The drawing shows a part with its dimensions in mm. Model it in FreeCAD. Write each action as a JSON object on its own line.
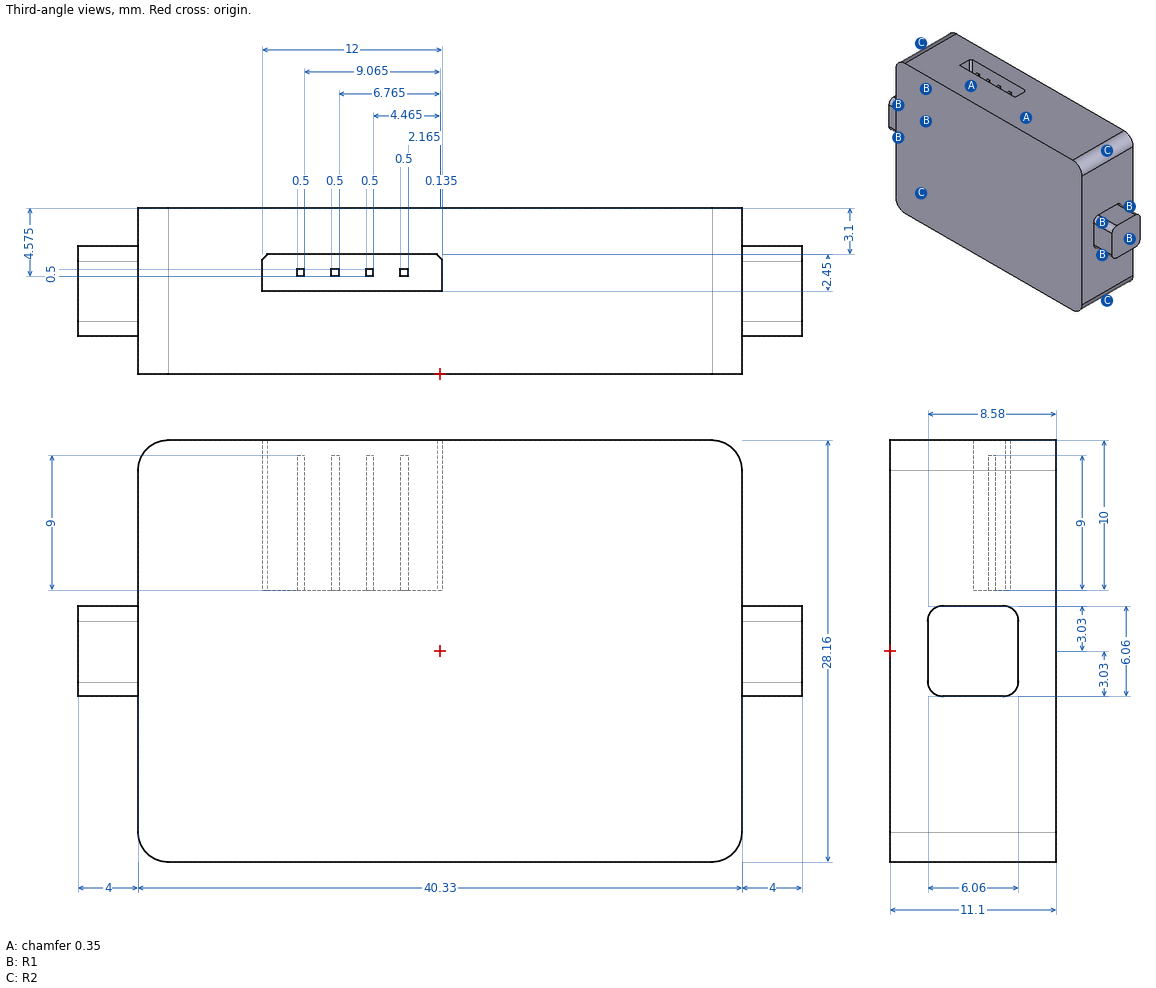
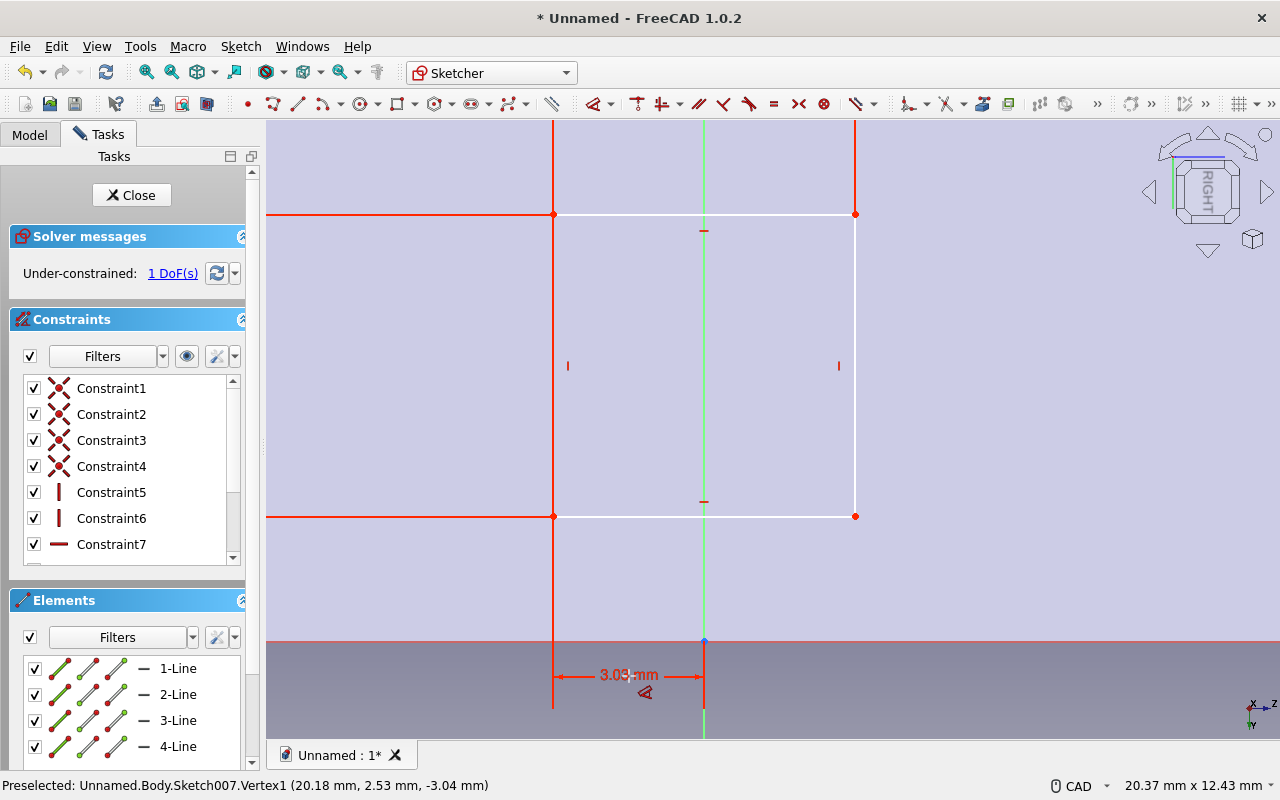
{"action": "left_click", "coordinate": [553, 215]}
{"action": "left_click", "coordinate": [519, 428]}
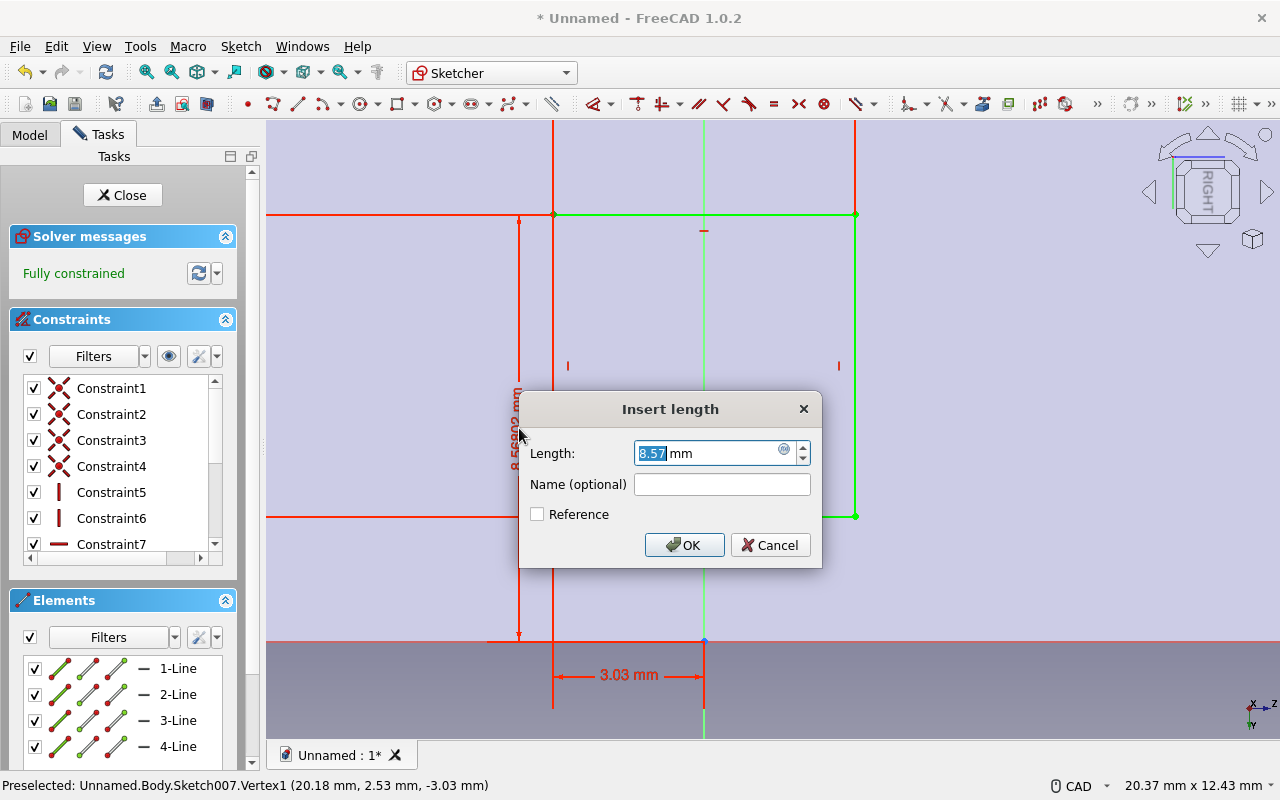
{"action": "type", "text": "8.58"}
{"action": "key", "text": "Return"}
{"action": "key", "text": "Escape"}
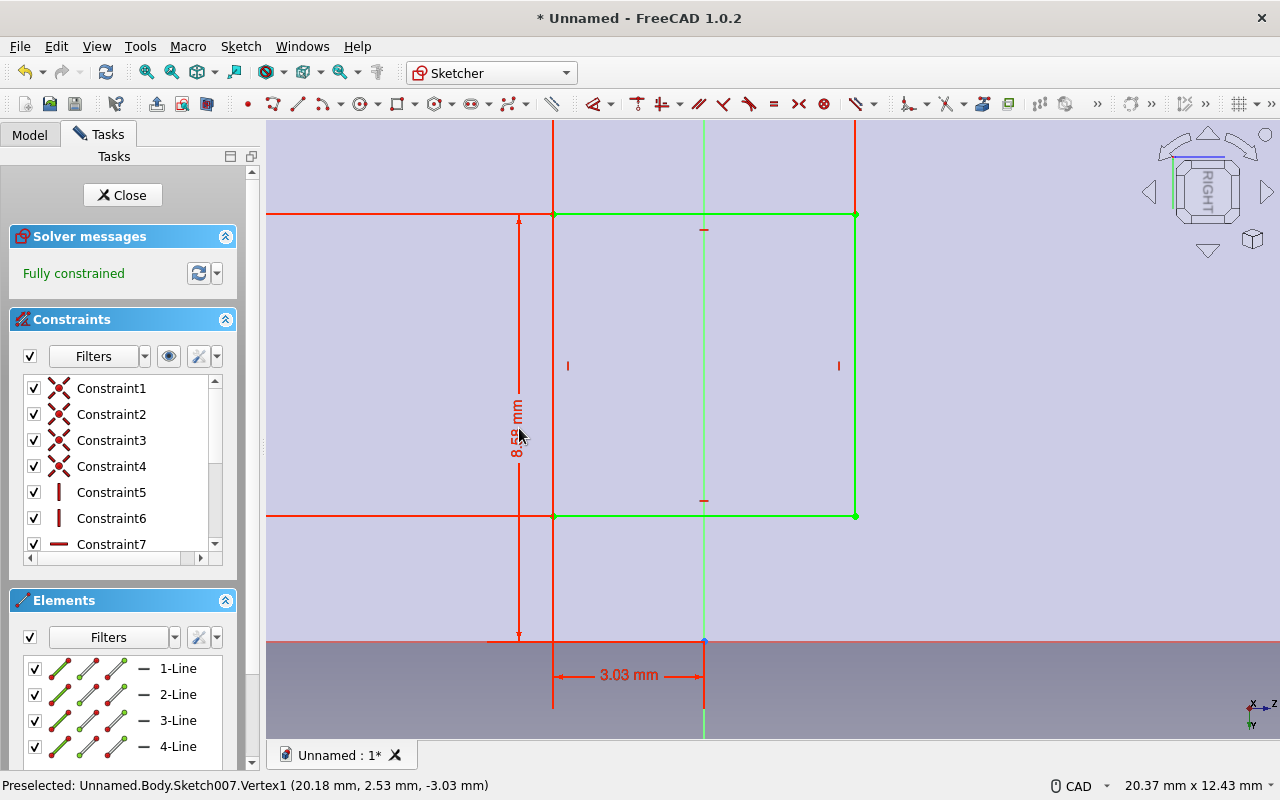
{"action": "left_click", "coordinate": [123, 195]}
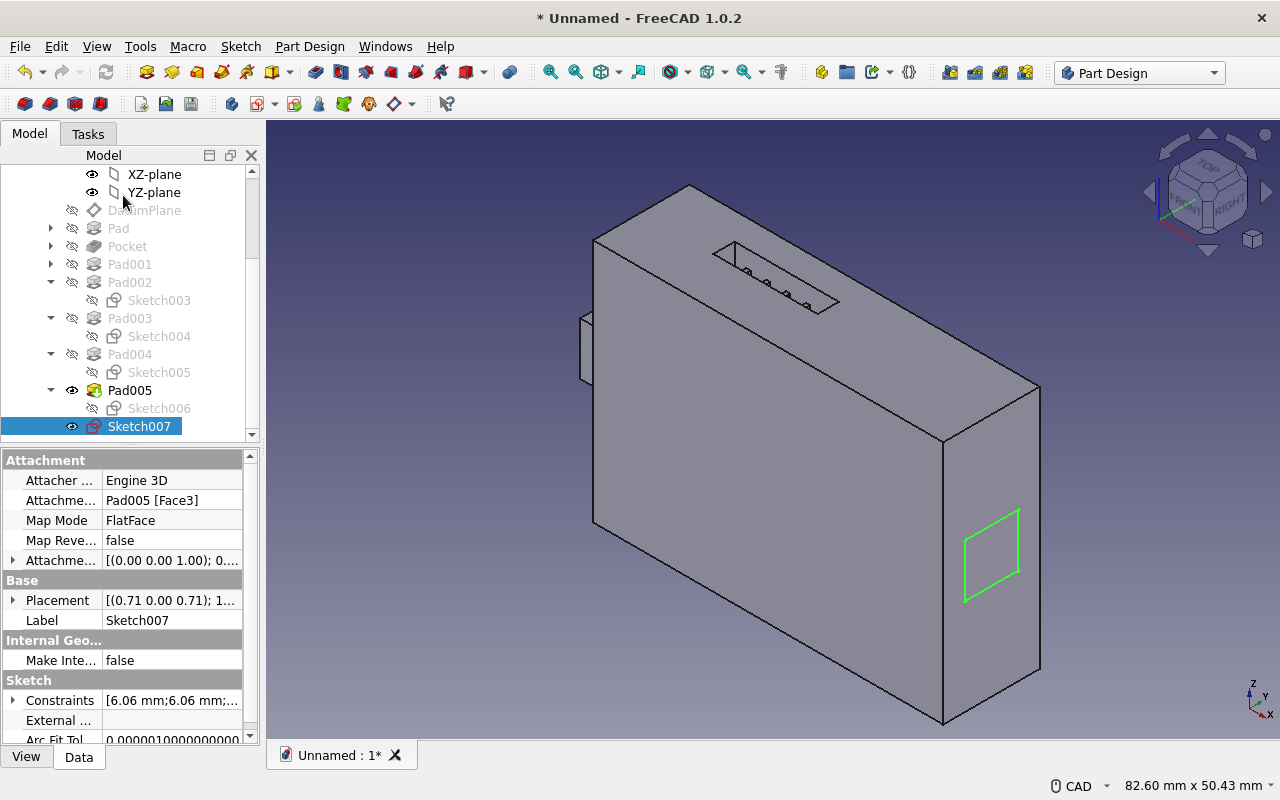
{"action": "left_click", "coordinate": [147, 72]}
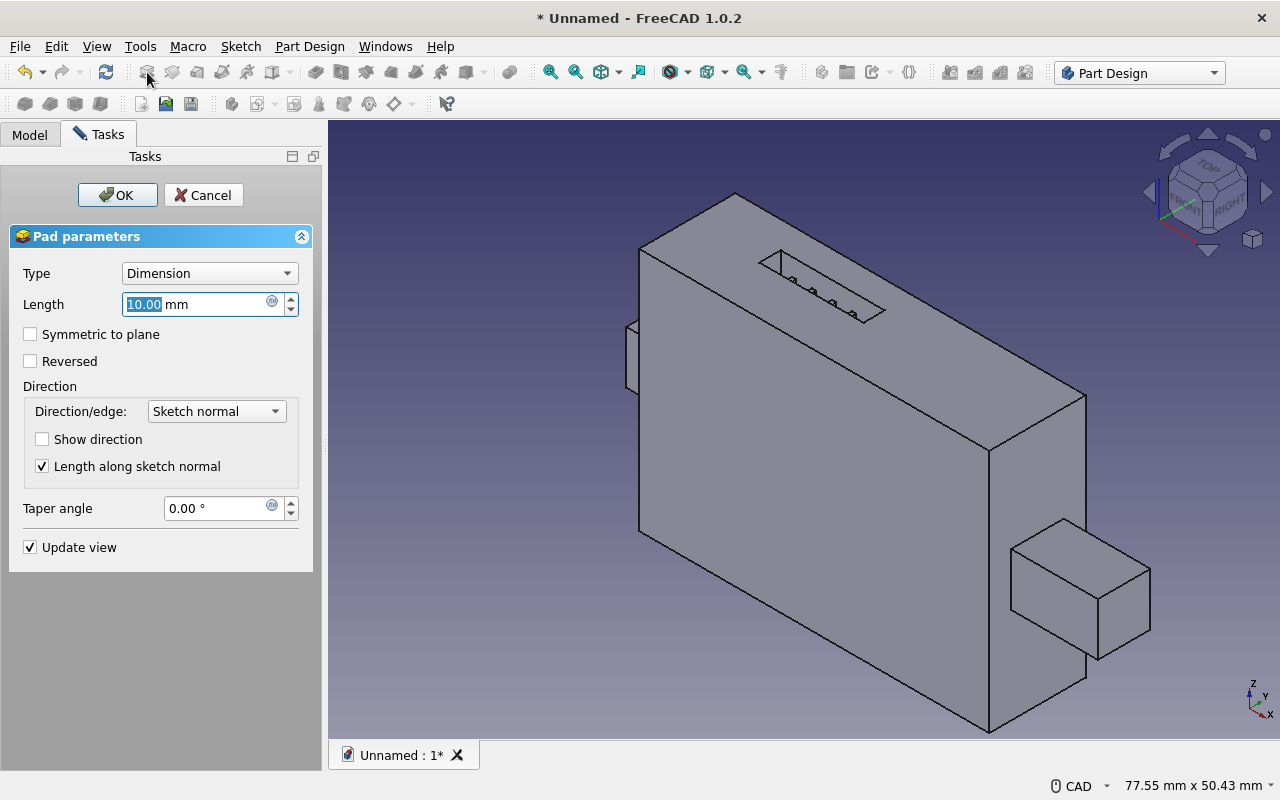
{"action": "type", "text": "4"}
{"action": "key", "text": "Tab"}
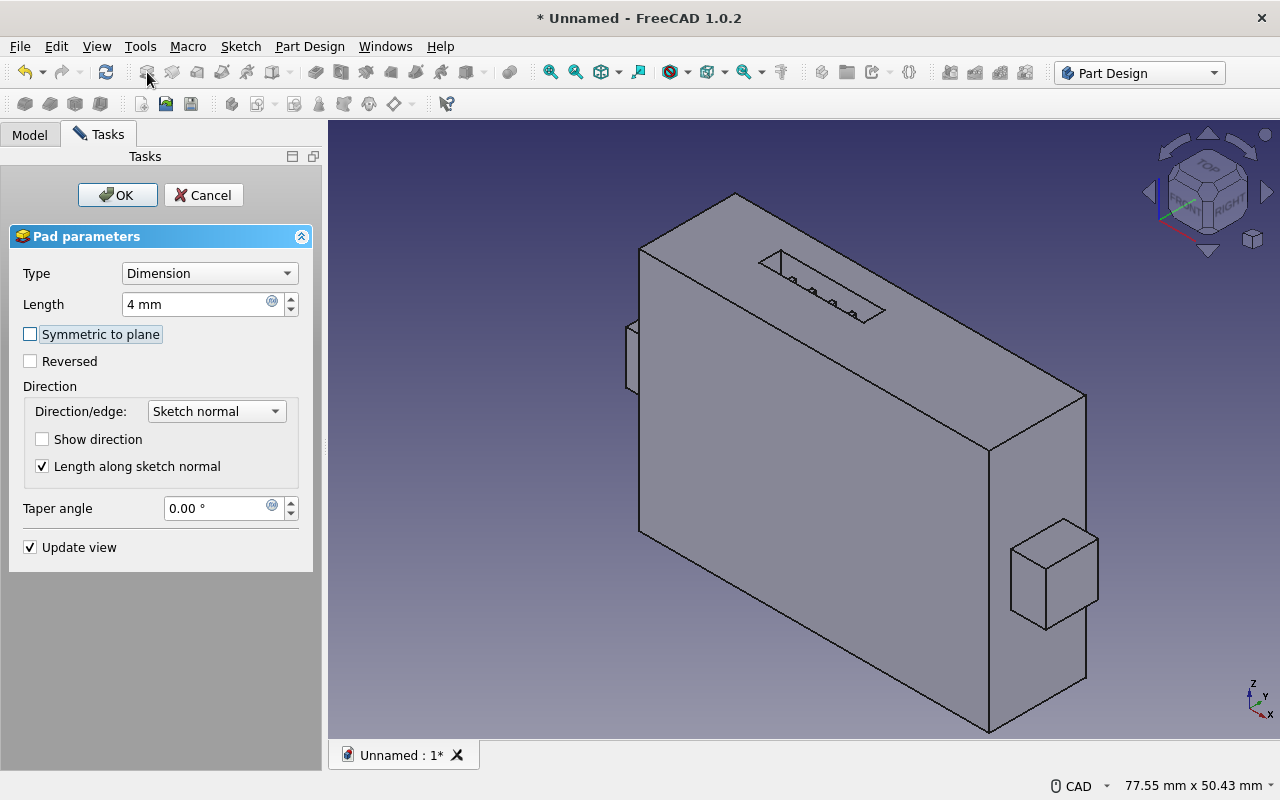
{"action": "left_click", "coordinate": [118, 195]}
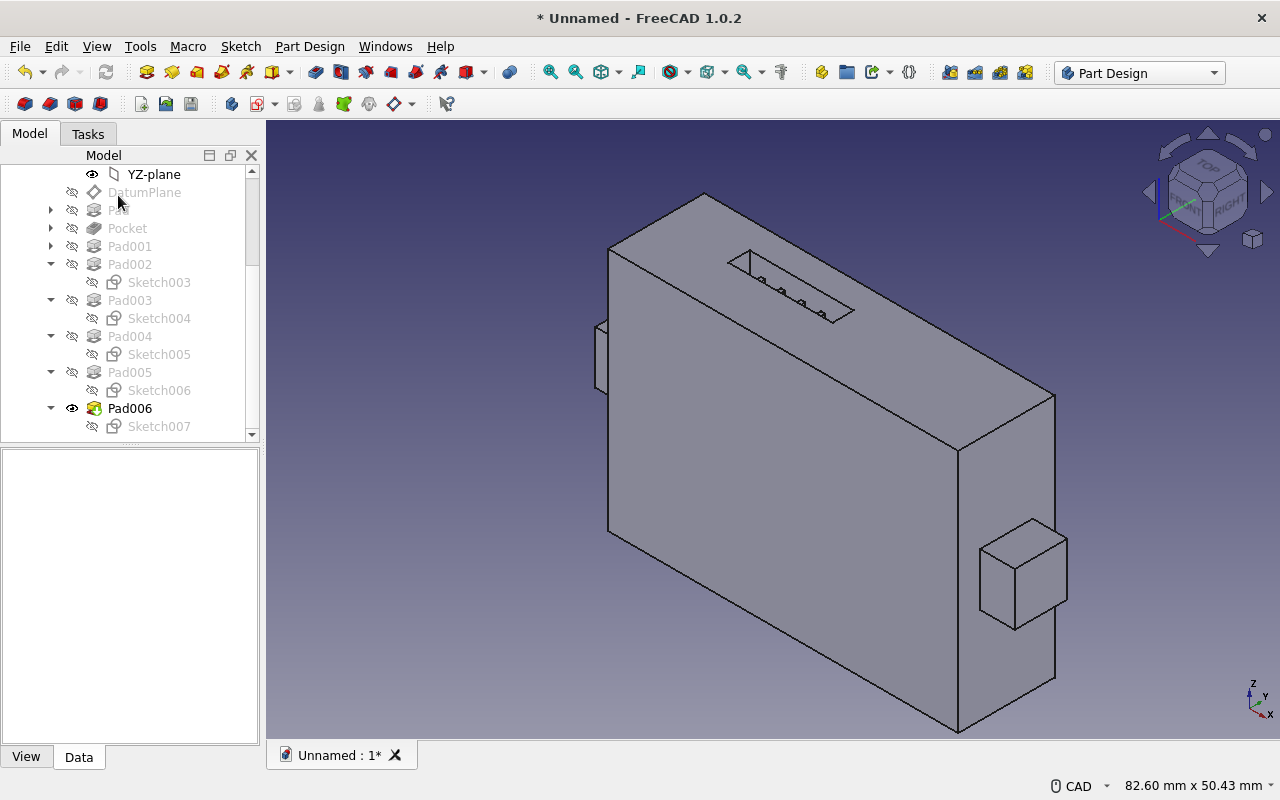
{"action": "left_click", "coordinate": [551, 72]}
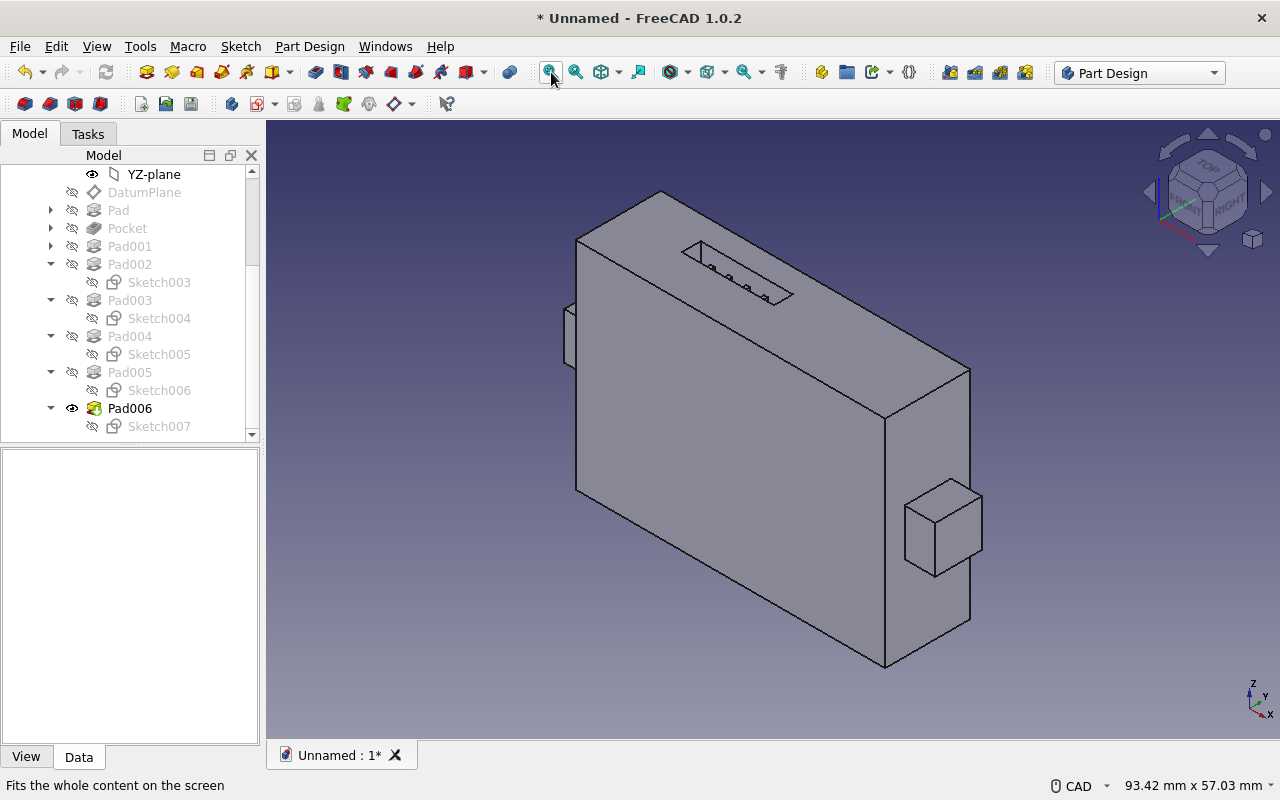
{"action": "key", "text": "2"}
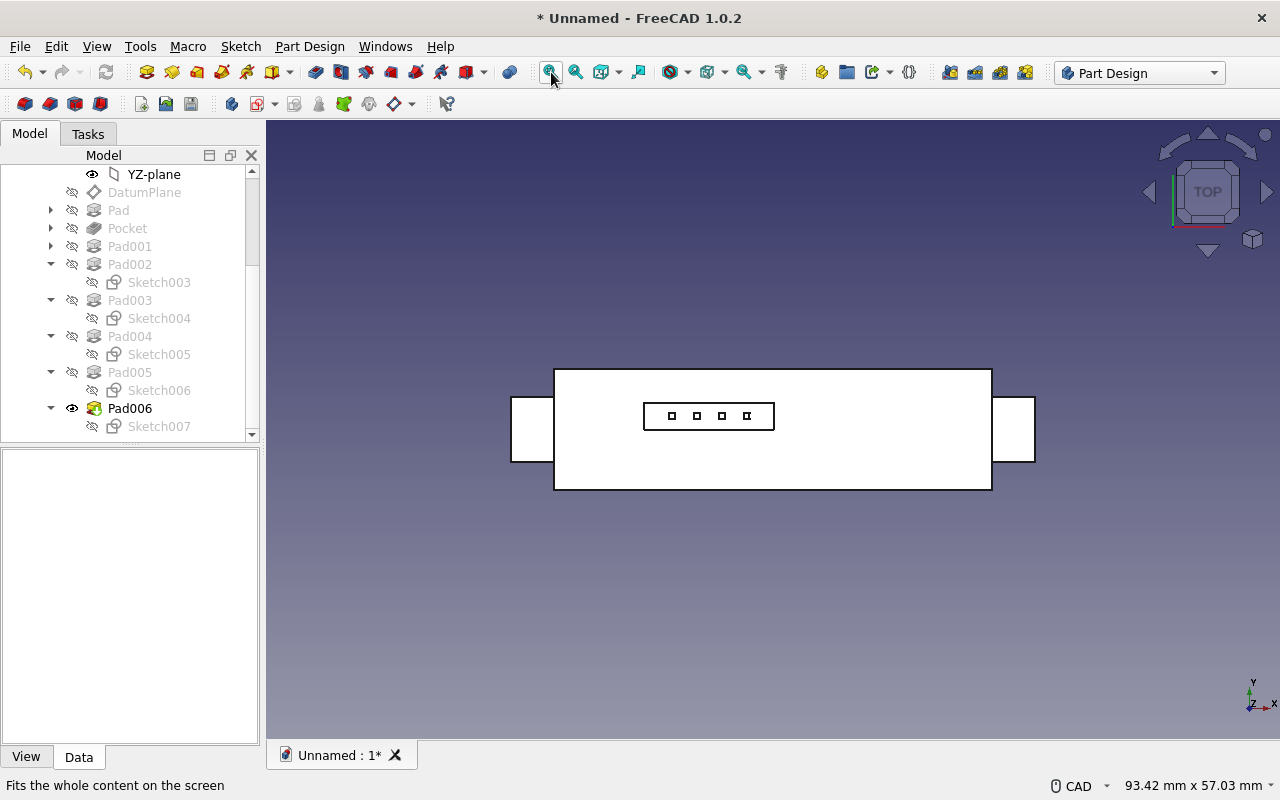
{"action": "key", "text": "0"}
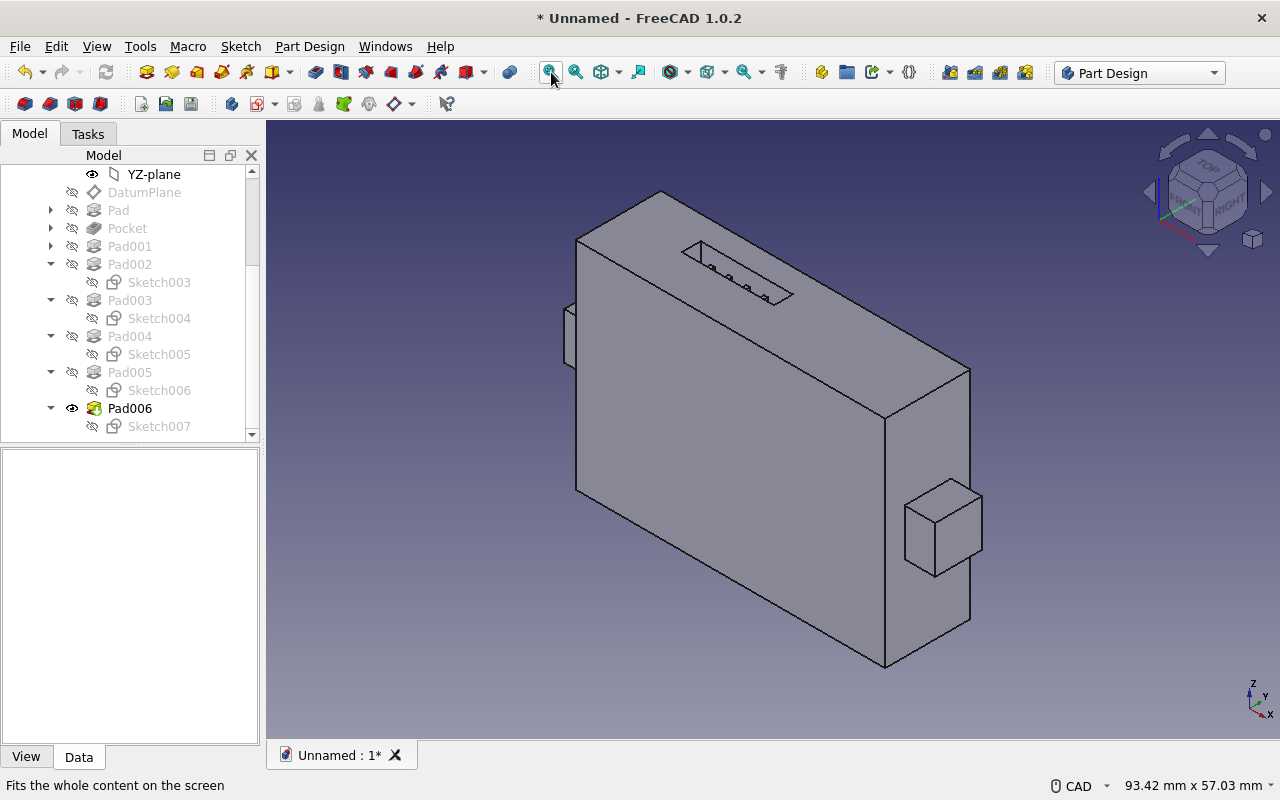
{"action": "key", "text": "1"}